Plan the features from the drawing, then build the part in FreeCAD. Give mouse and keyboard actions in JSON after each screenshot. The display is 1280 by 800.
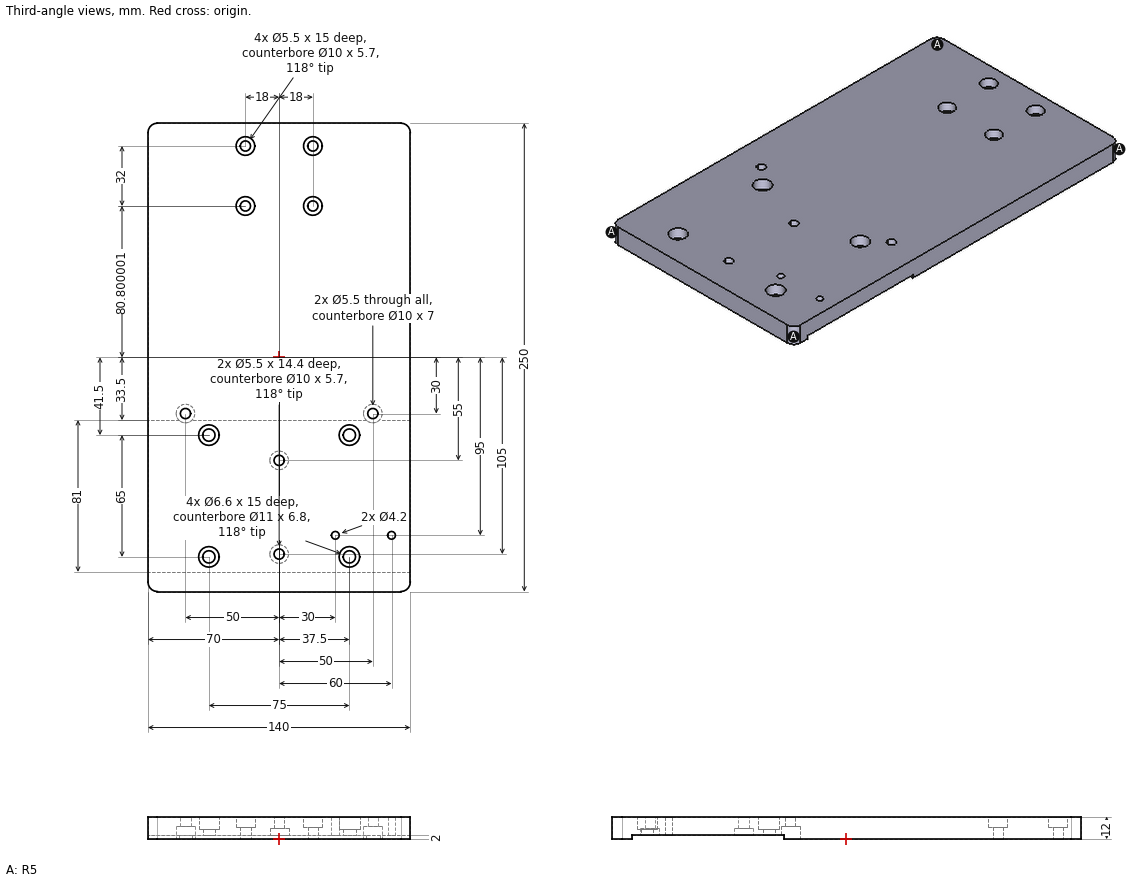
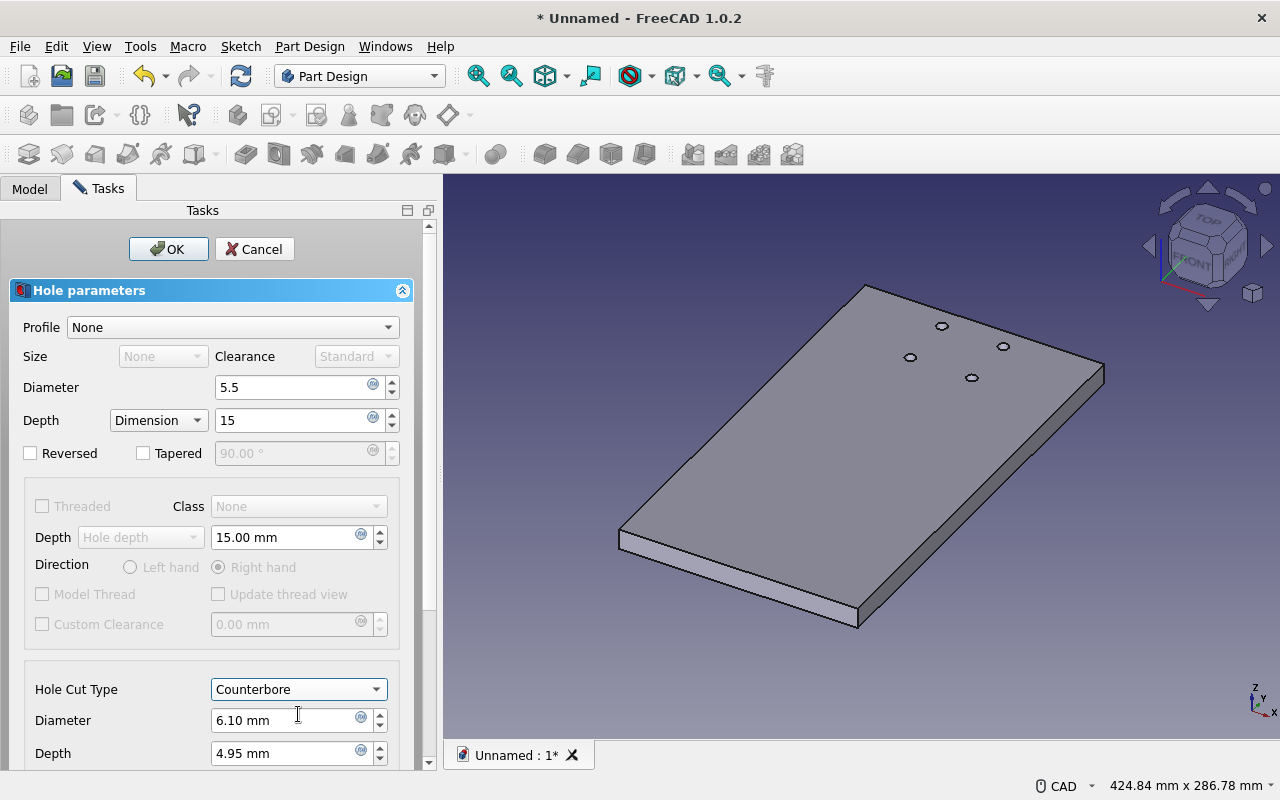
{"action": "triple_click", "coordinate": [292, 720]}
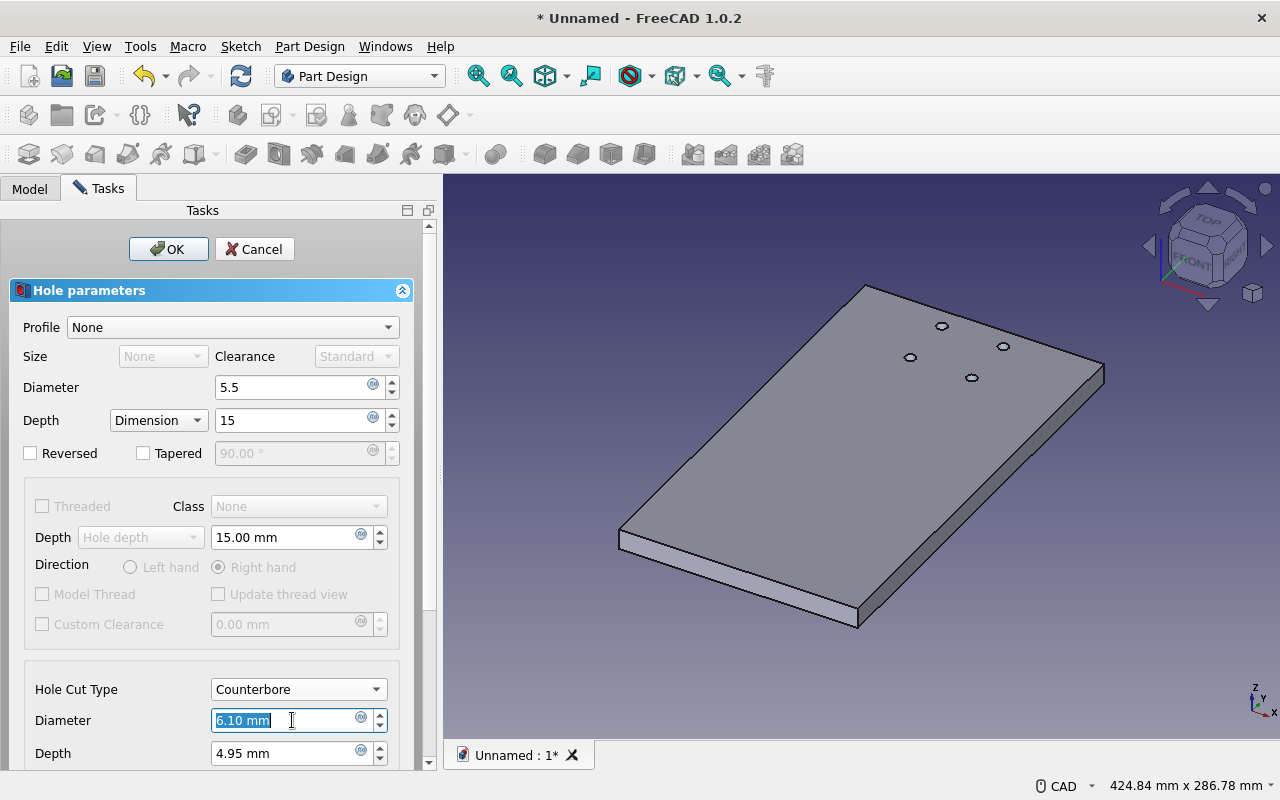
{"action": "type", "text": "10"}
{"action": "key", "text": "Tab"}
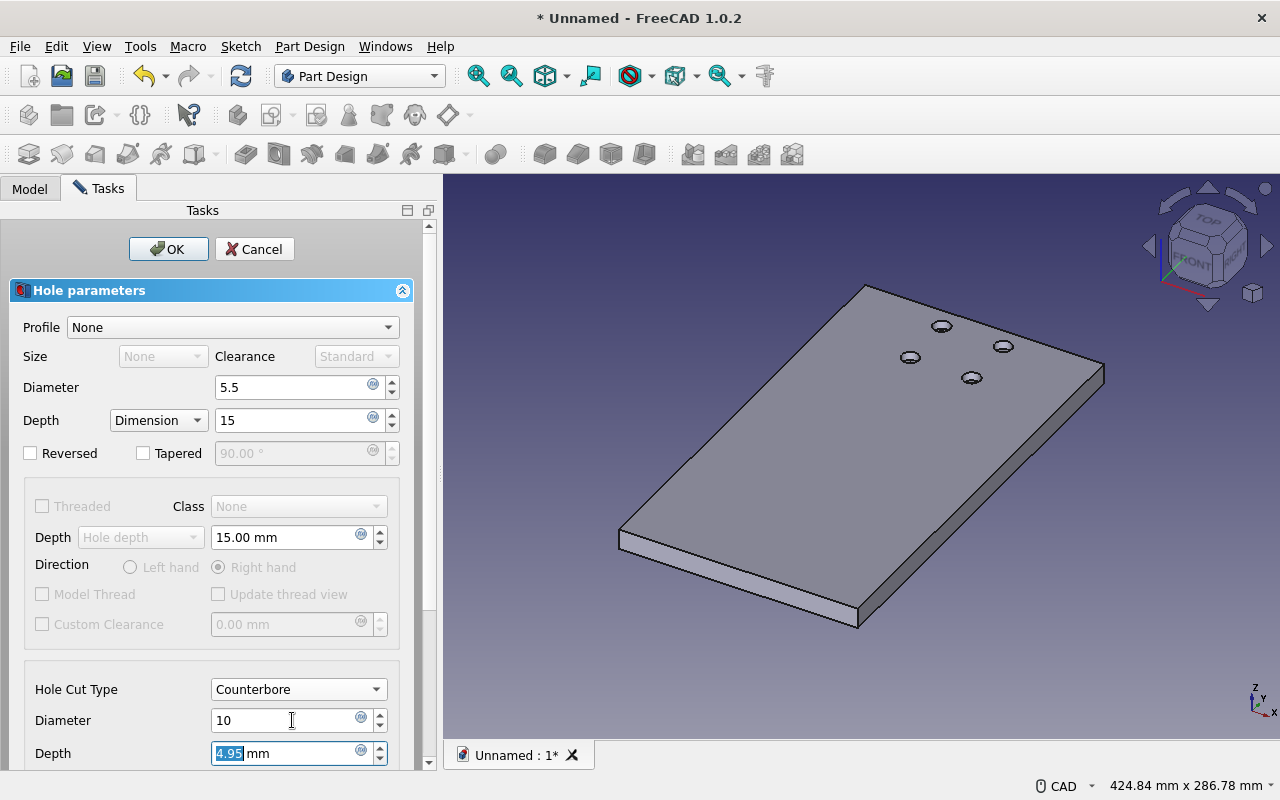
{"action": "type", "text": "5.7"}
{"action": "key", "text": "Tab"}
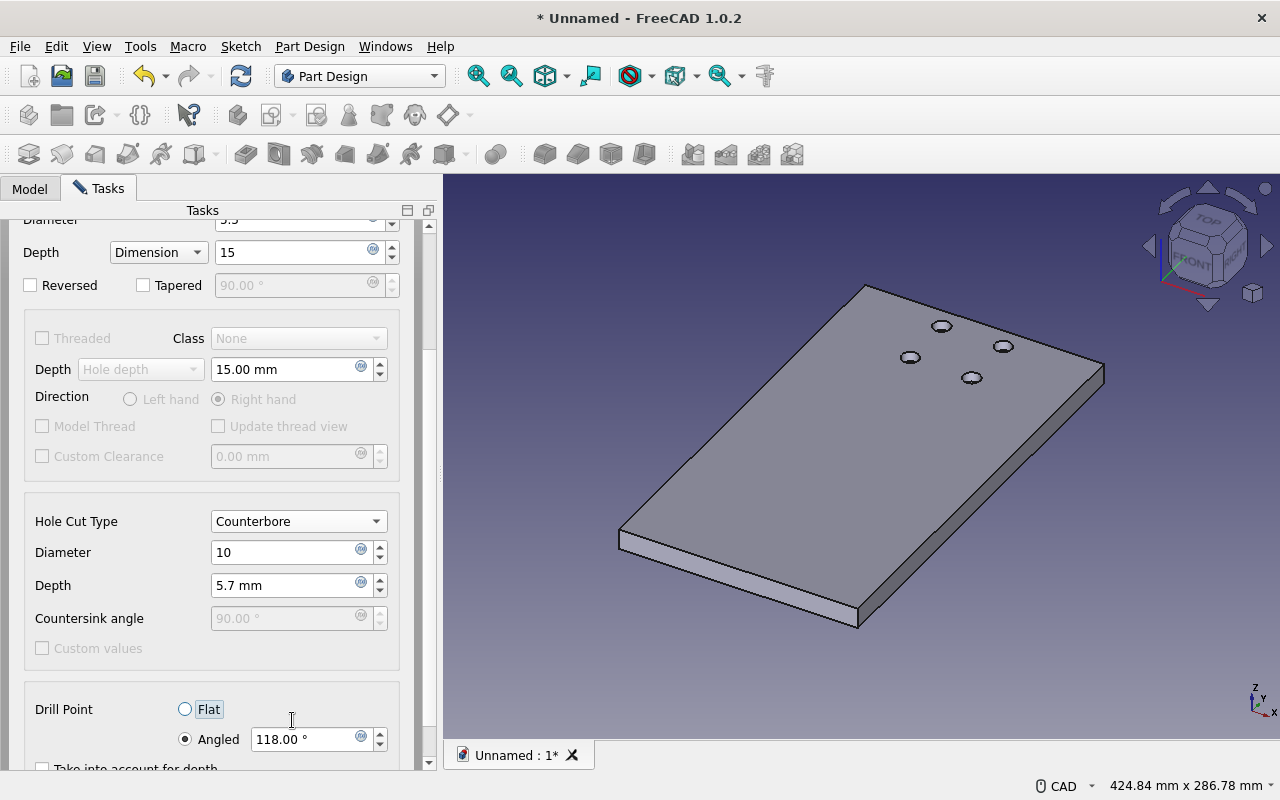
{"action": "scroll", "coordinate": [429, 495], "scroll_direction": "up", "scroll_amount": 4}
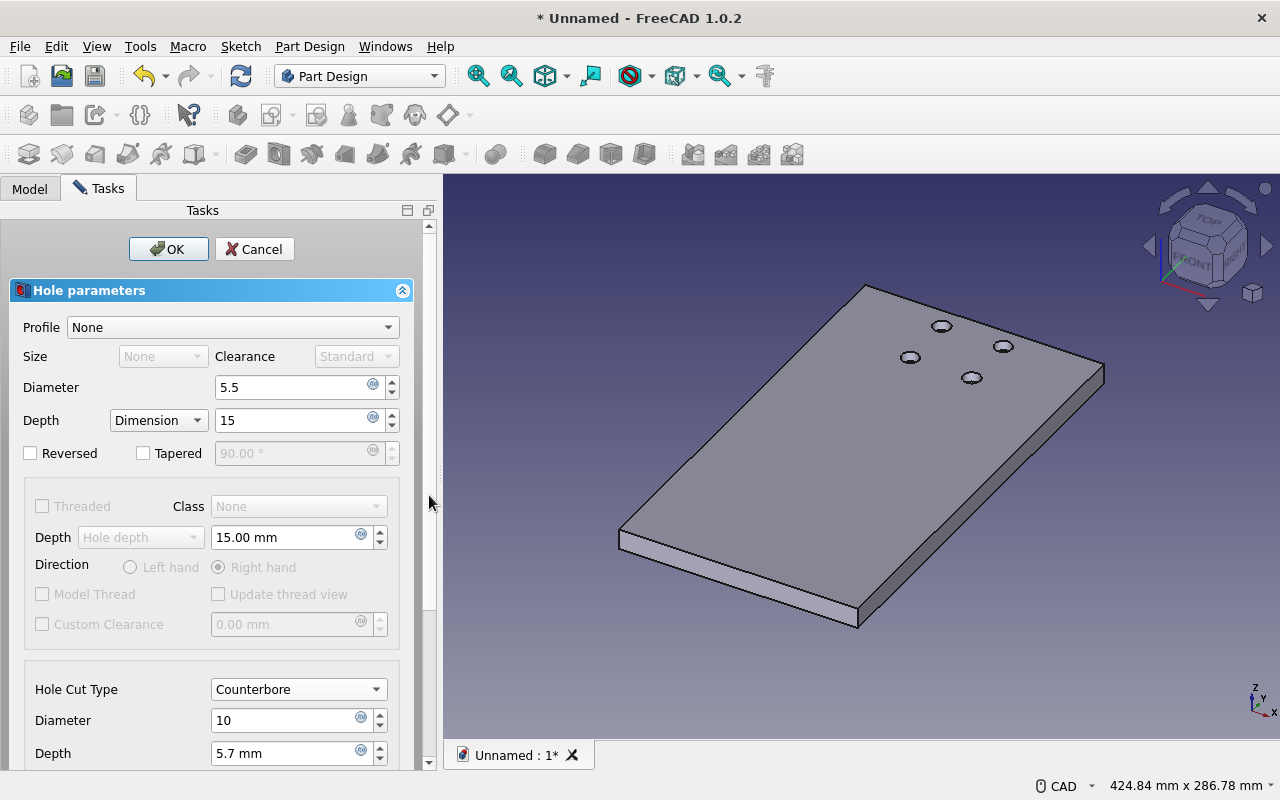
{"action": "left_click", "coordinate": [169, 249]}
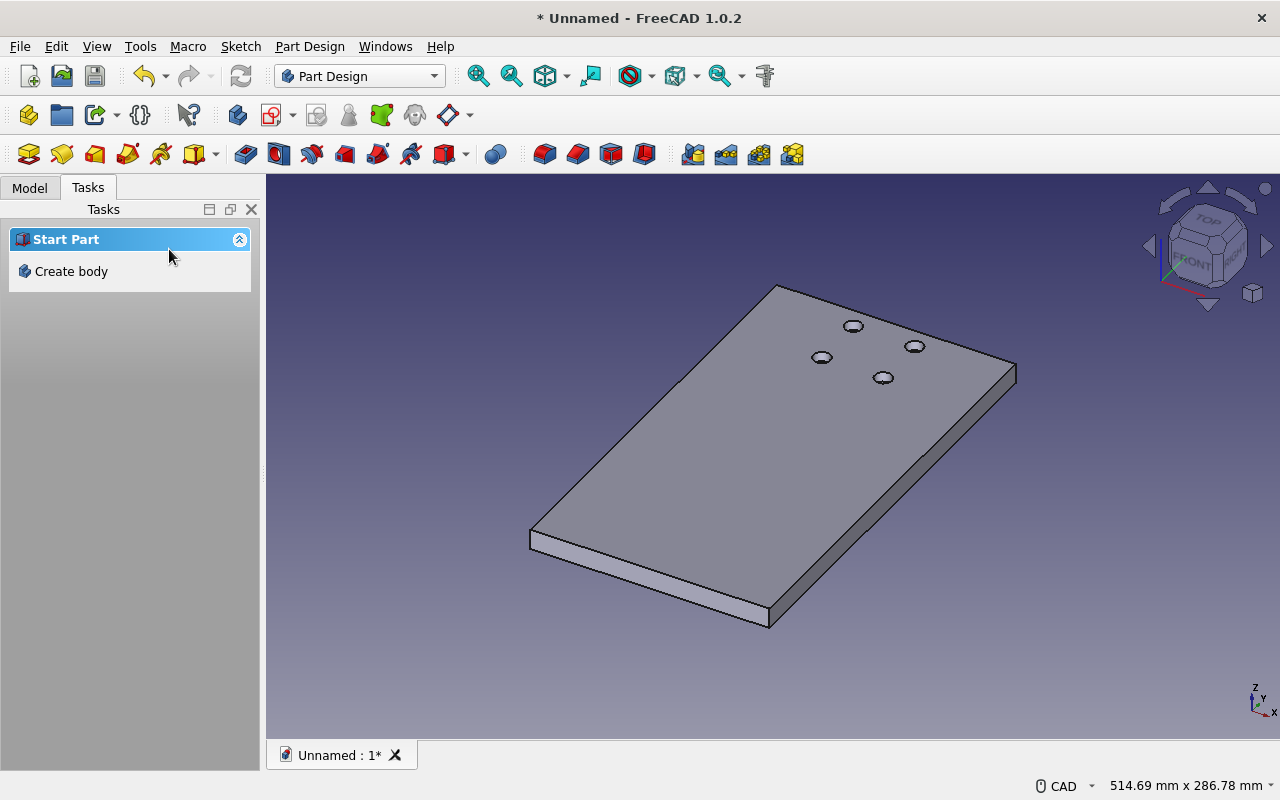
{"action": "left_click", "coordinate": [773, 446]}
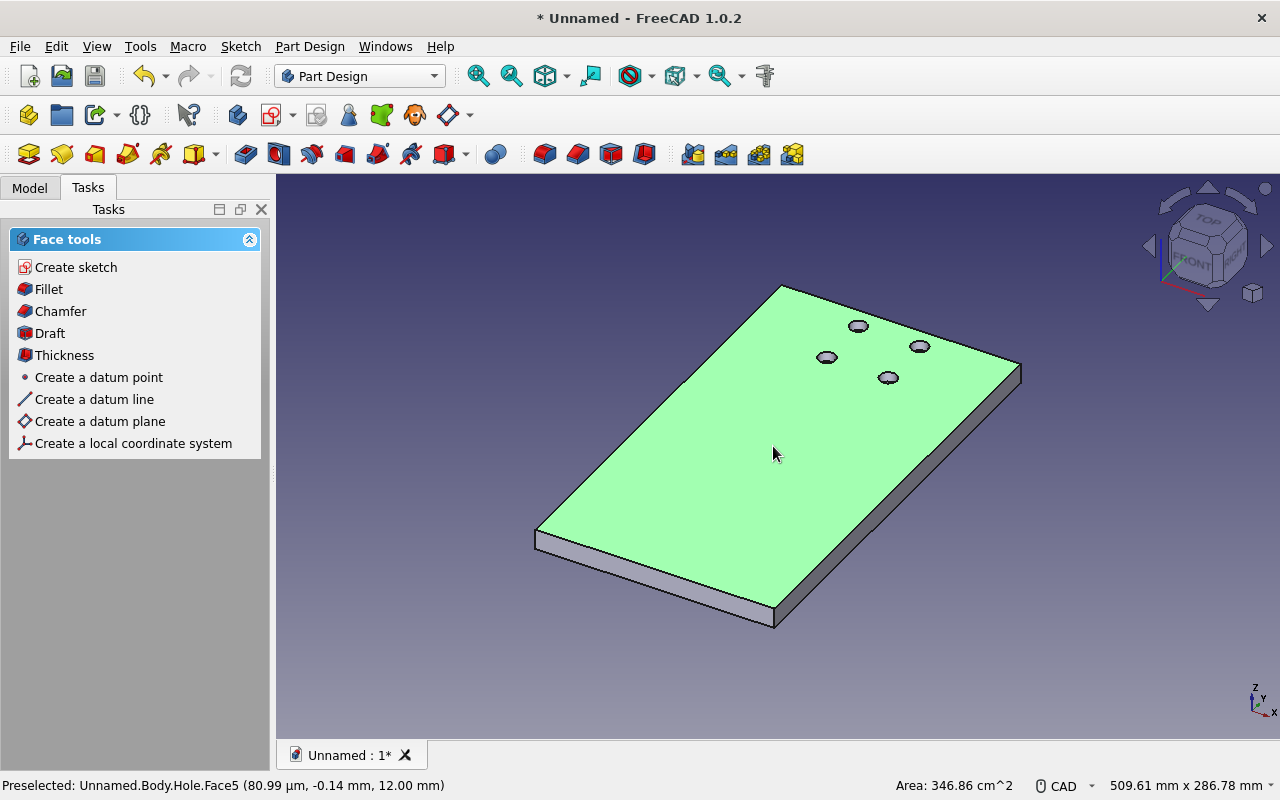
{"action": "left_click", "coordinate": [270, 116]}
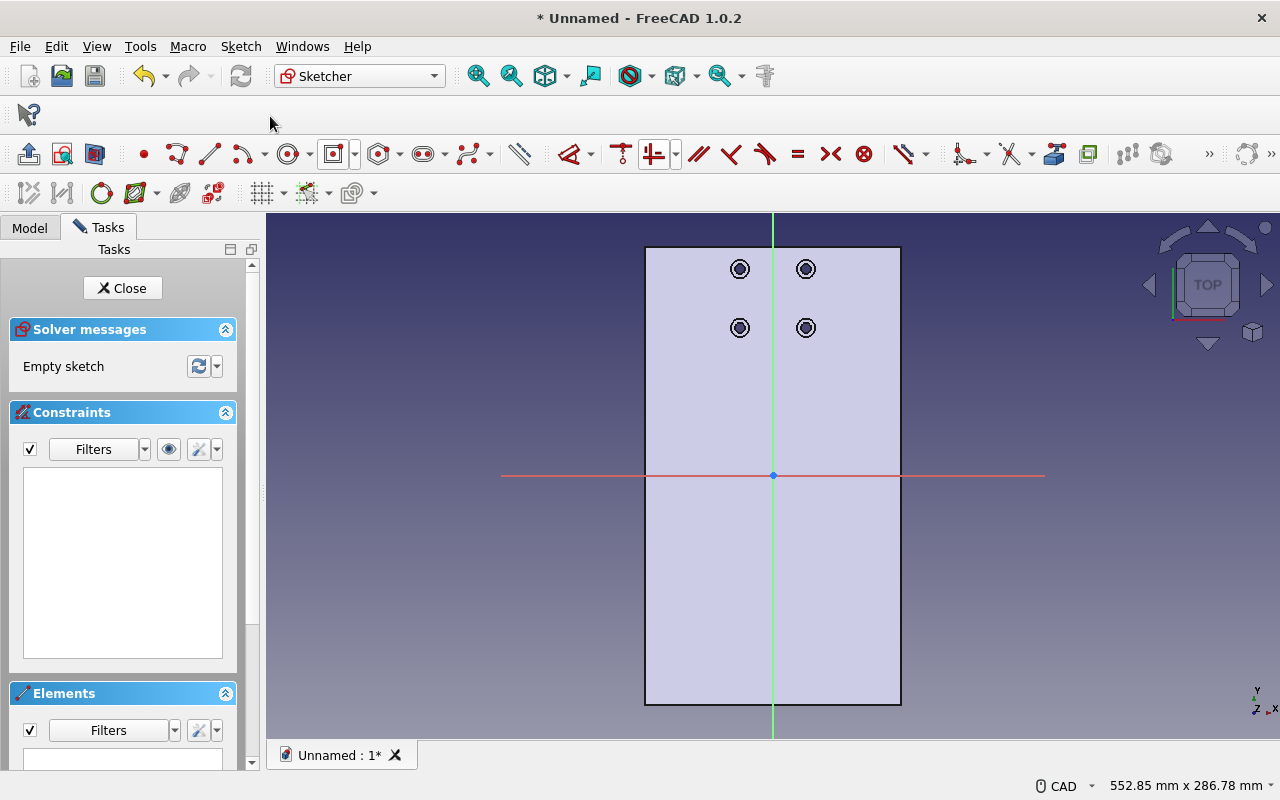
{"action": "scroll", "coordinate": [912, 711], "scroll_direction": "up", "scroll_amount": 2}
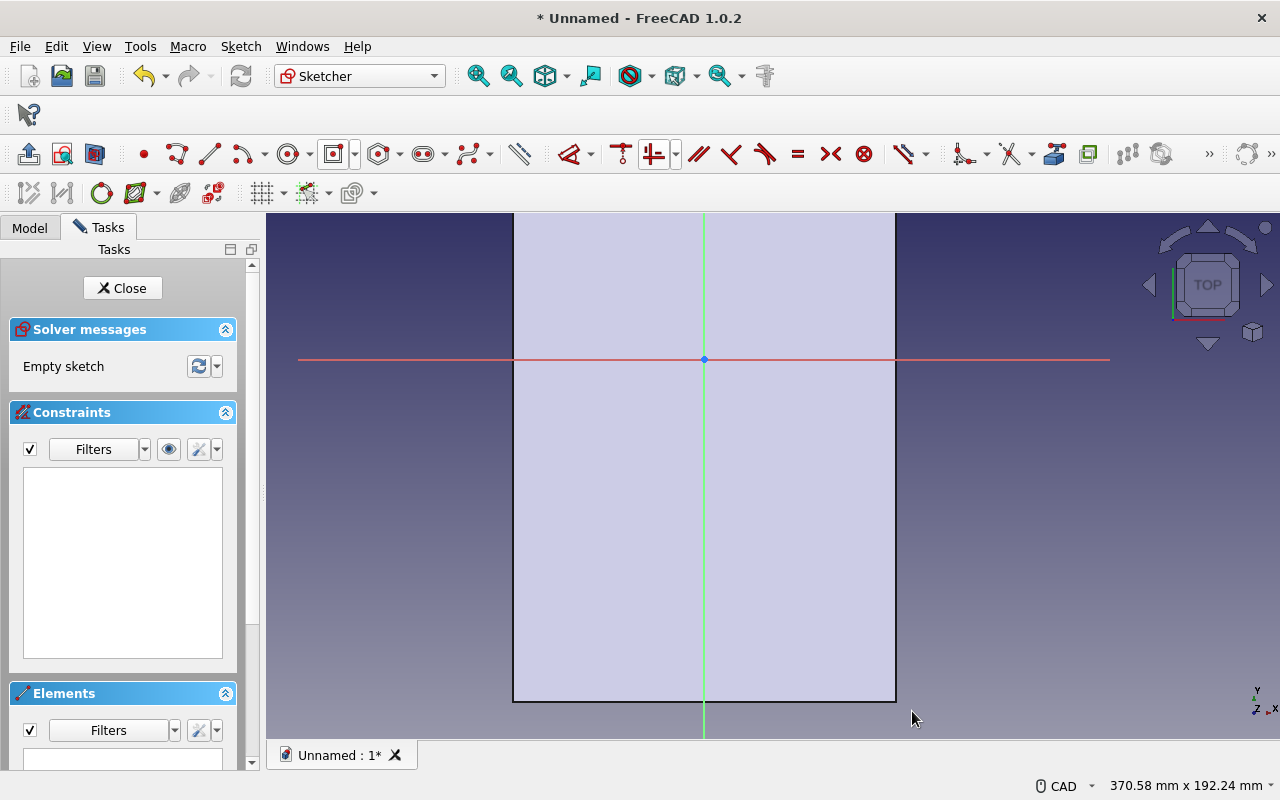
{"action": "left_click", "coordinate": [288, 154]}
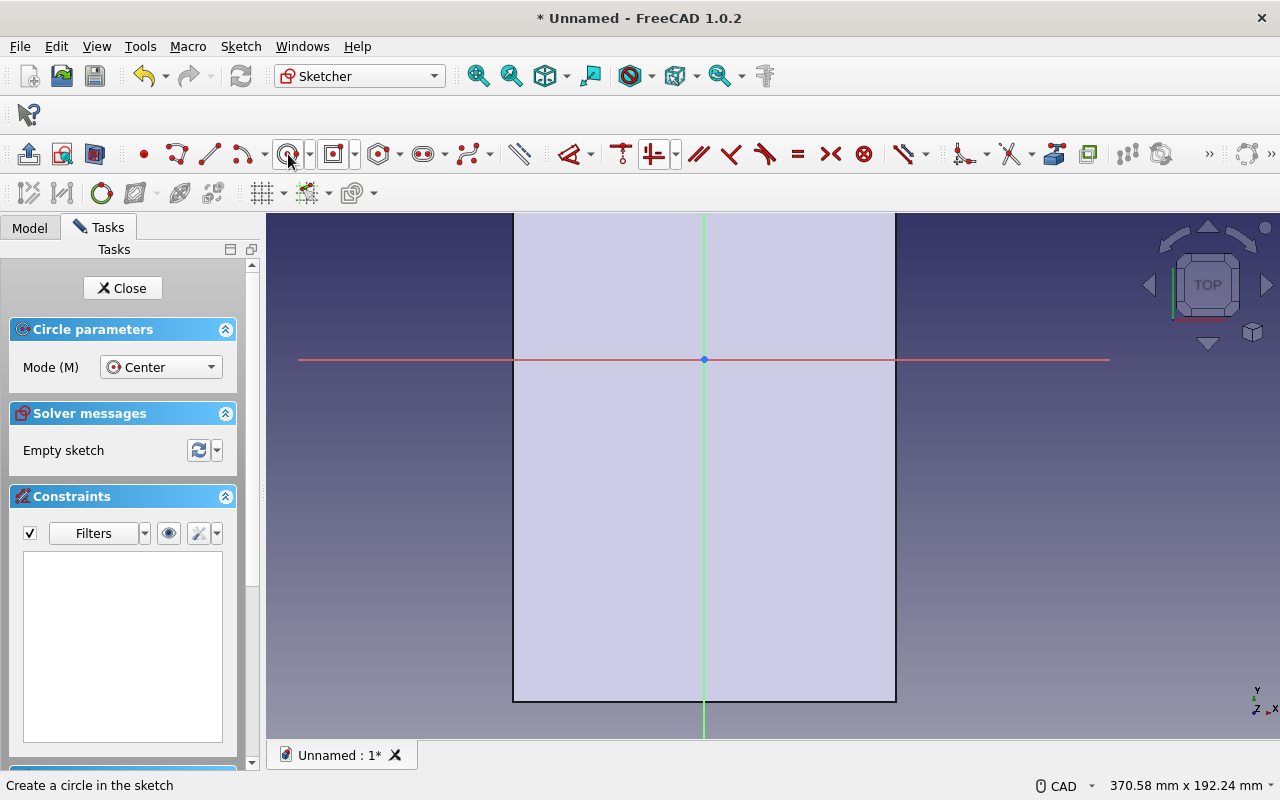
{"action": "scroll", "coordinate": [807, 651], "scroll_direction": "up", "scroll_amount": 5}